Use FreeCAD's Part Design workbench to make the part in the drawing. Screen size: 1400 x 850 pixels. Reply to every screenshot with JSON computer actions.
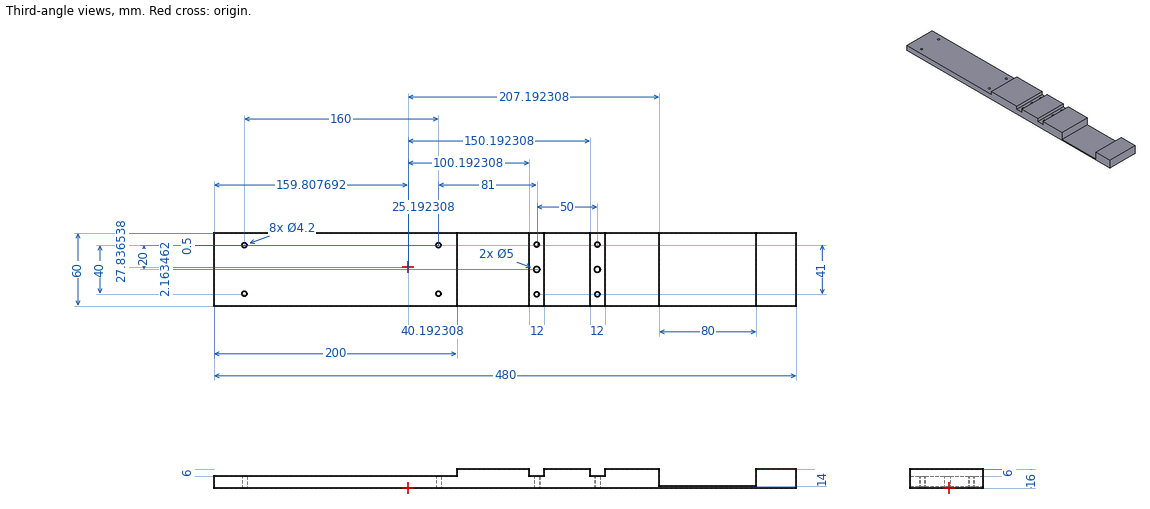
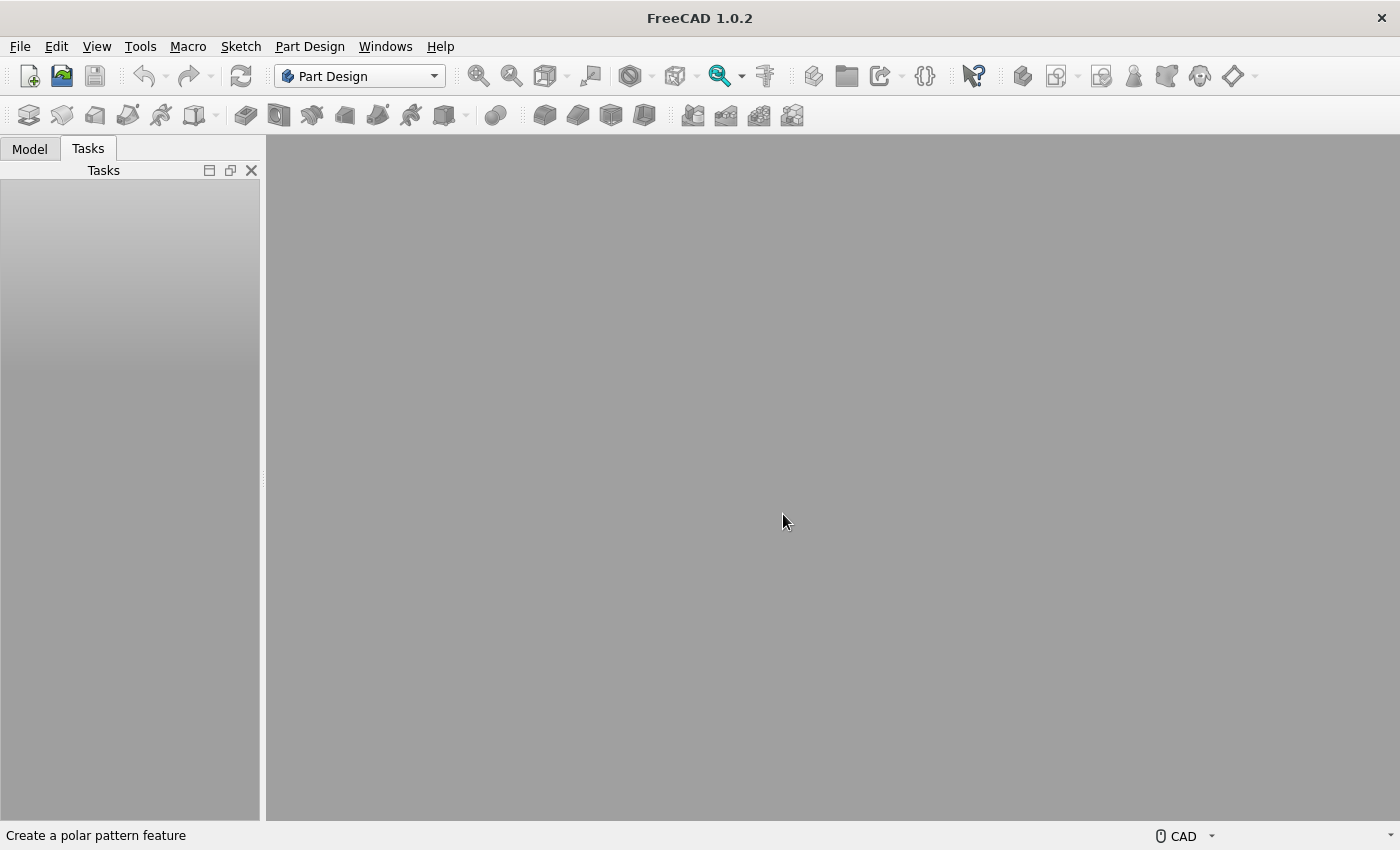
{"action": "left_click", "coordinate": [29, 76]}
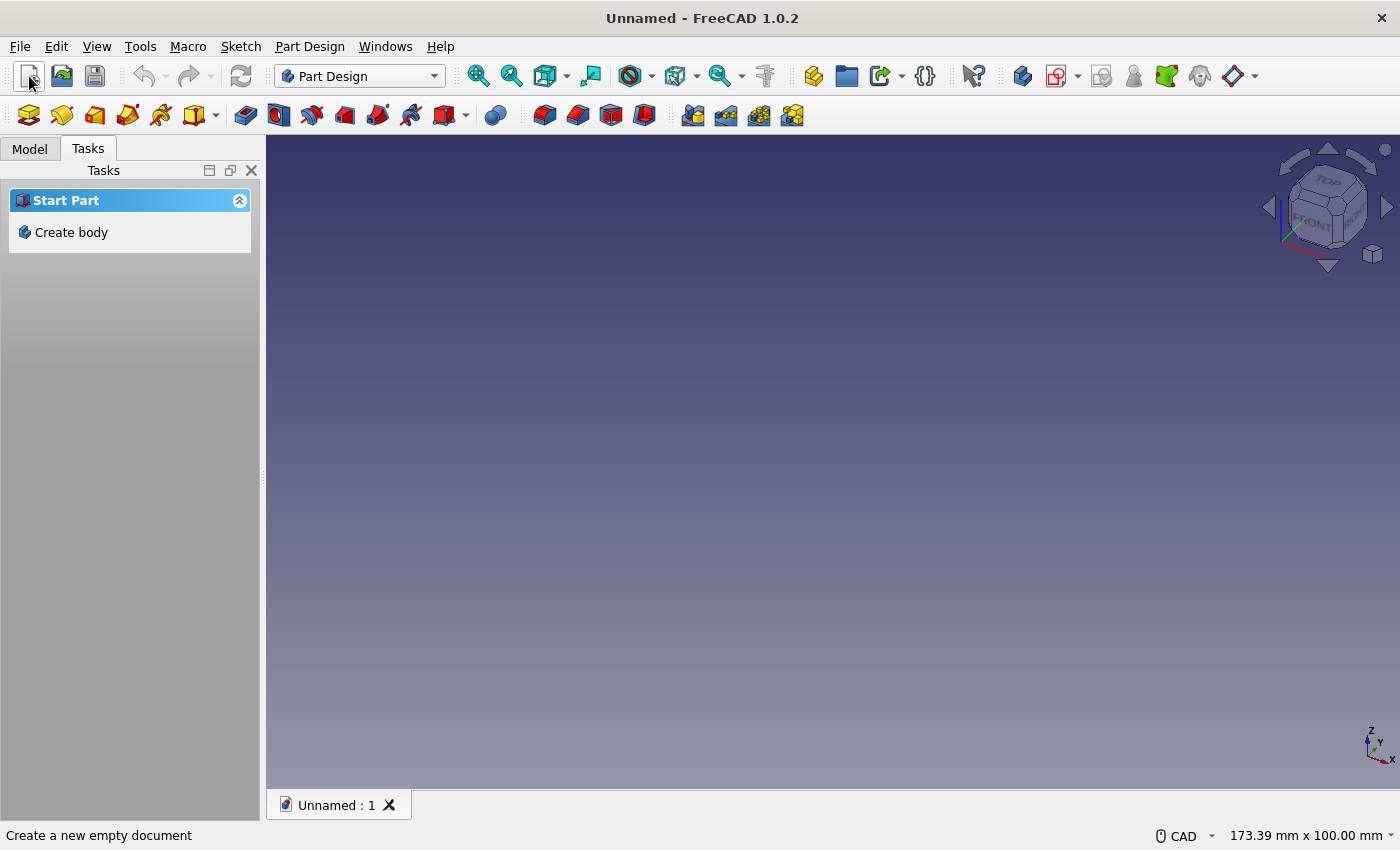
{"action": "left_click", "coordinate": [1056, 76]}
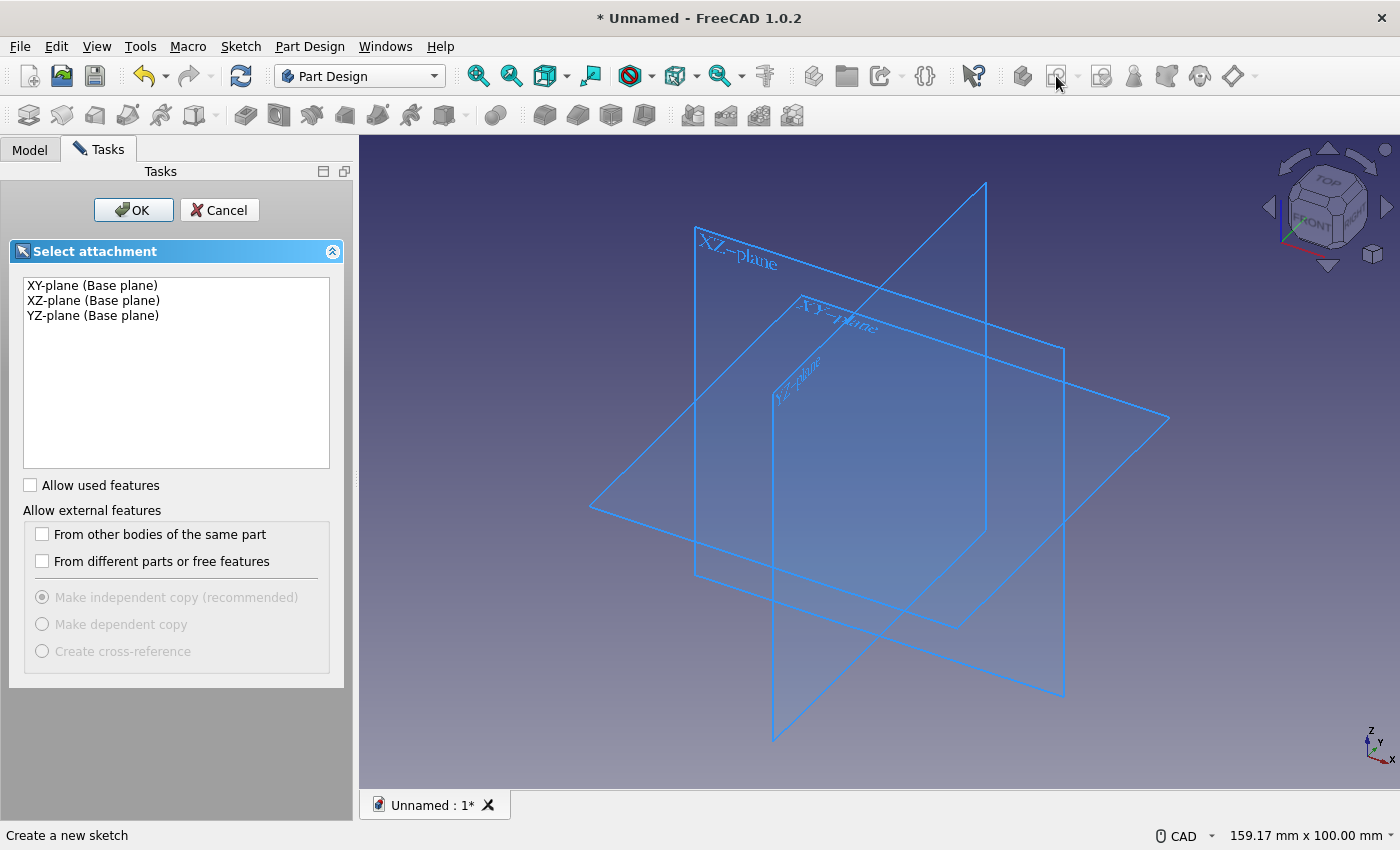
{"action": "left_click", "coordinate": [84, 286]}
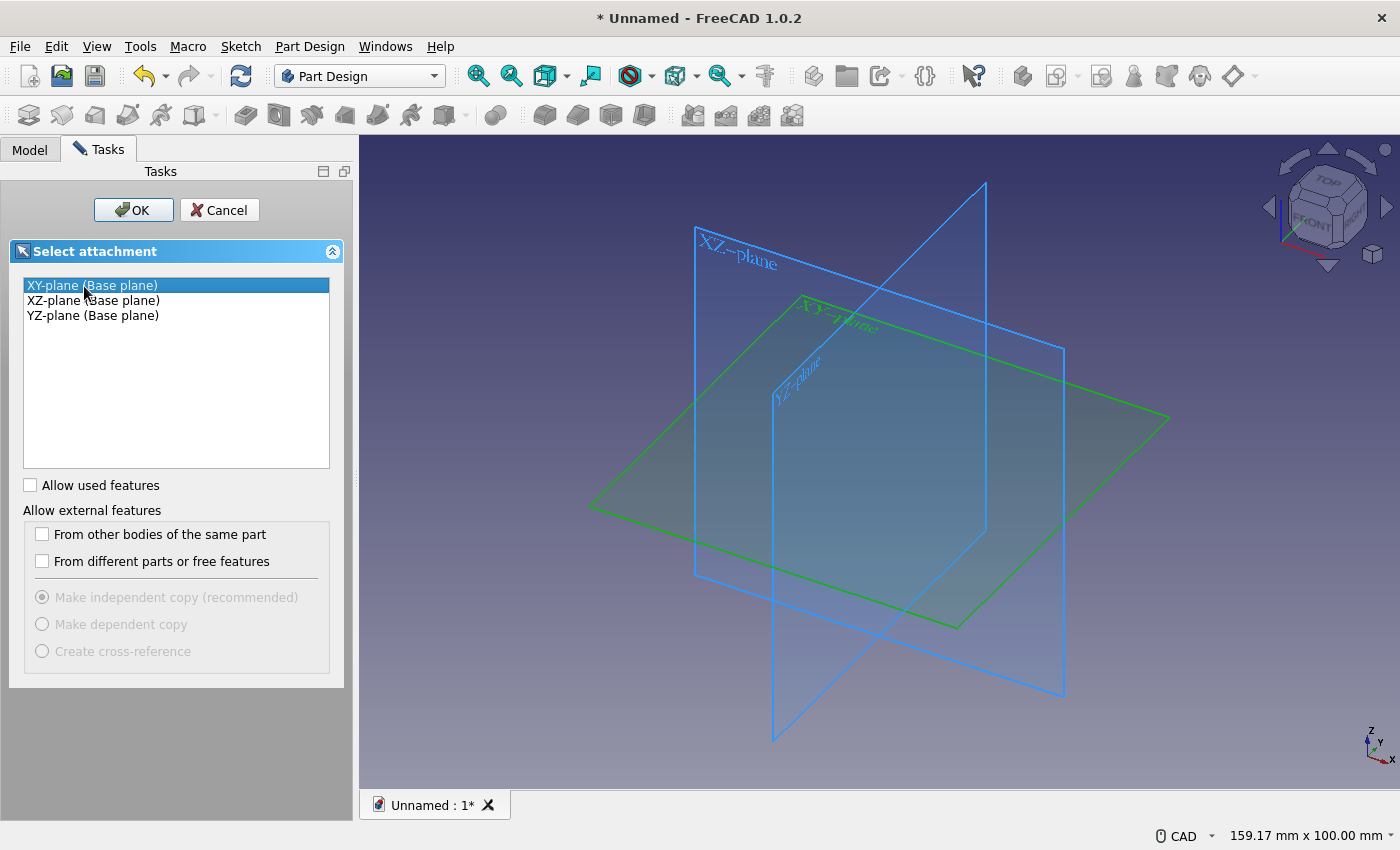
{"action": "left_click", "coordinate": [134, 210]}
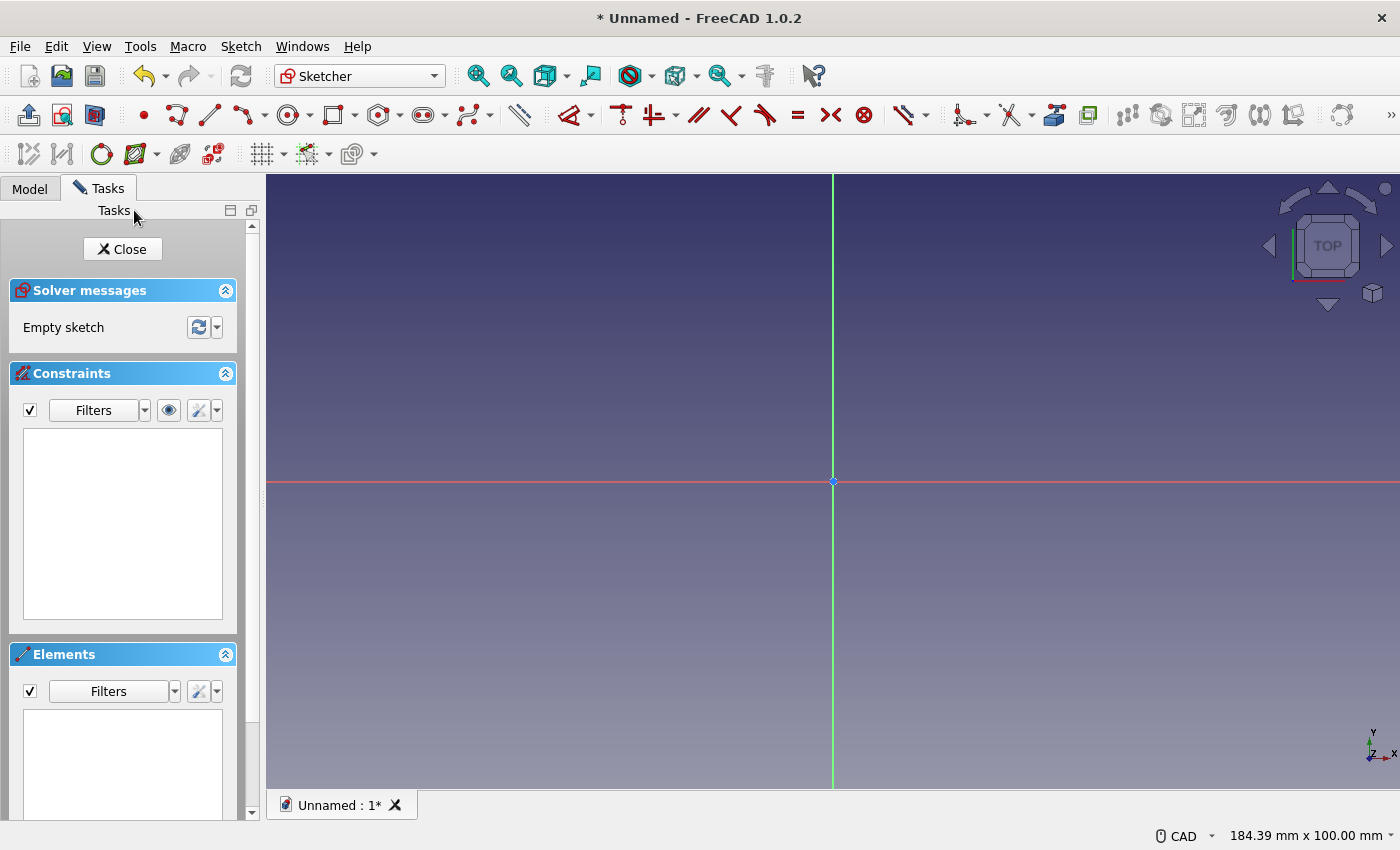
{"action": "scroll", "coordinate": [581, 477], "scroll_direction": "down", "scroll_amount": 7}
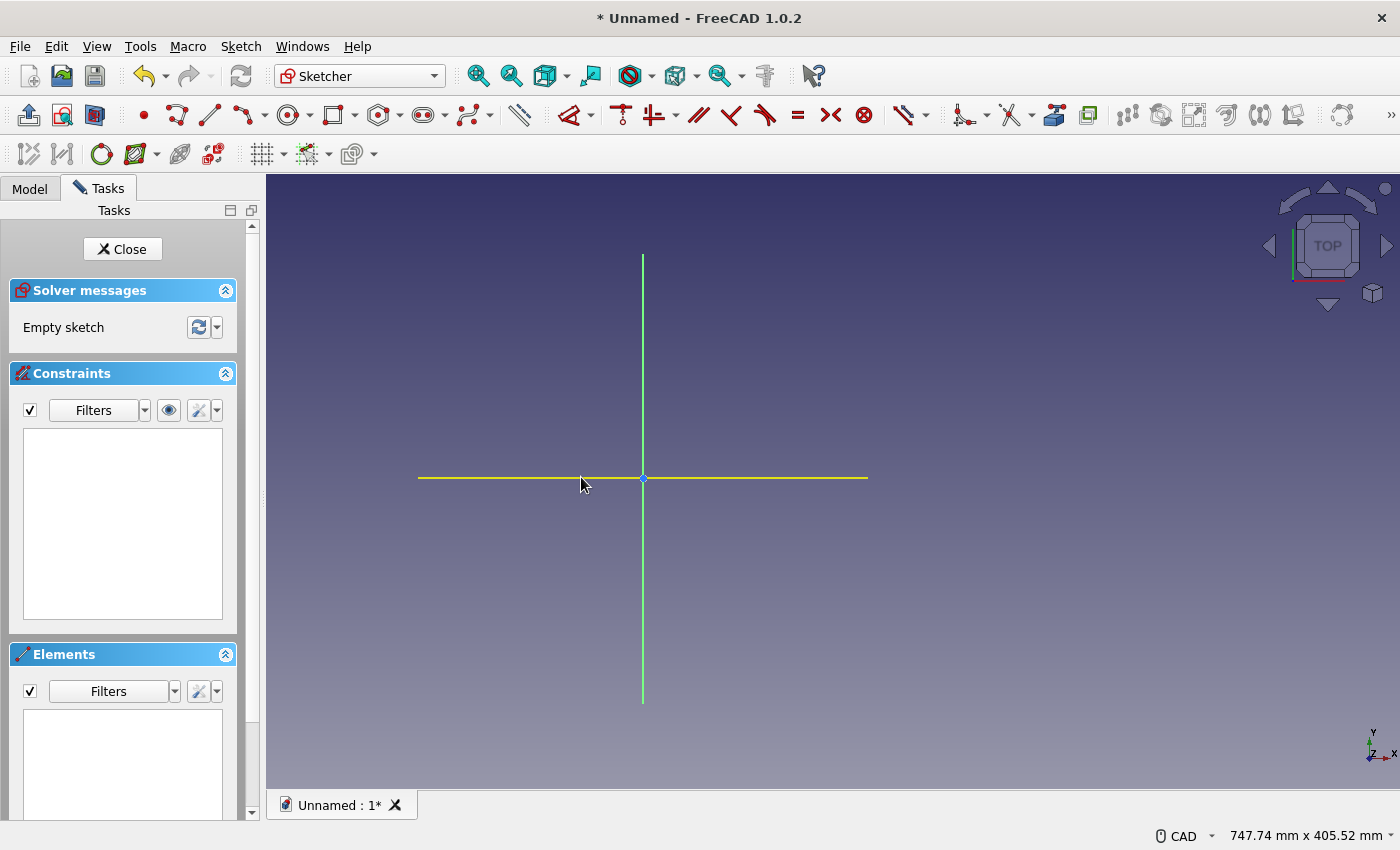
{"action": "left_click", "coordinate": [332, 116]}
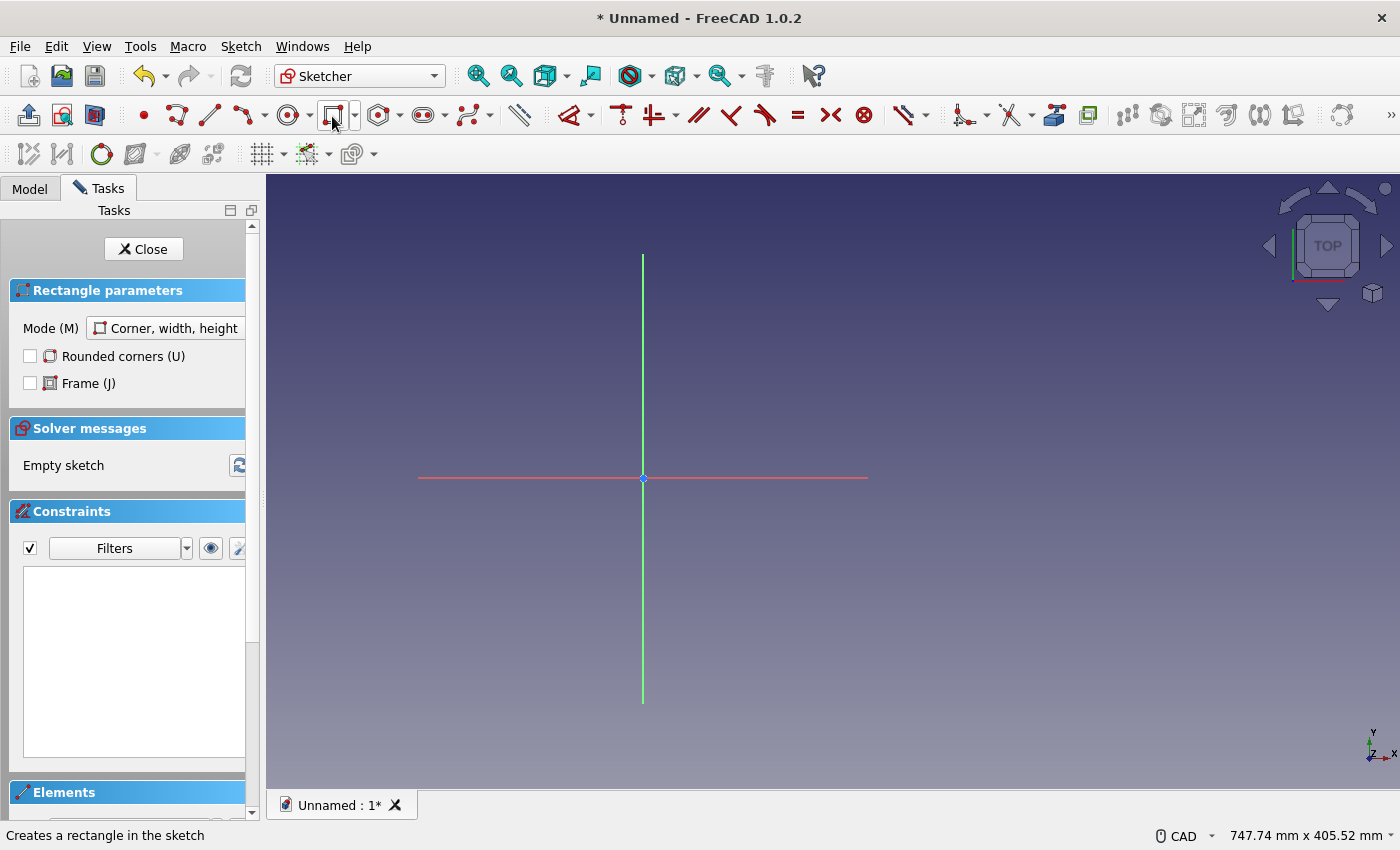
{"action": "left_click", "coordinate": [401, 436]}
{"action": "left_click", "coordinate": [1129, 527]}
{"action": "key", "text": "Escape"}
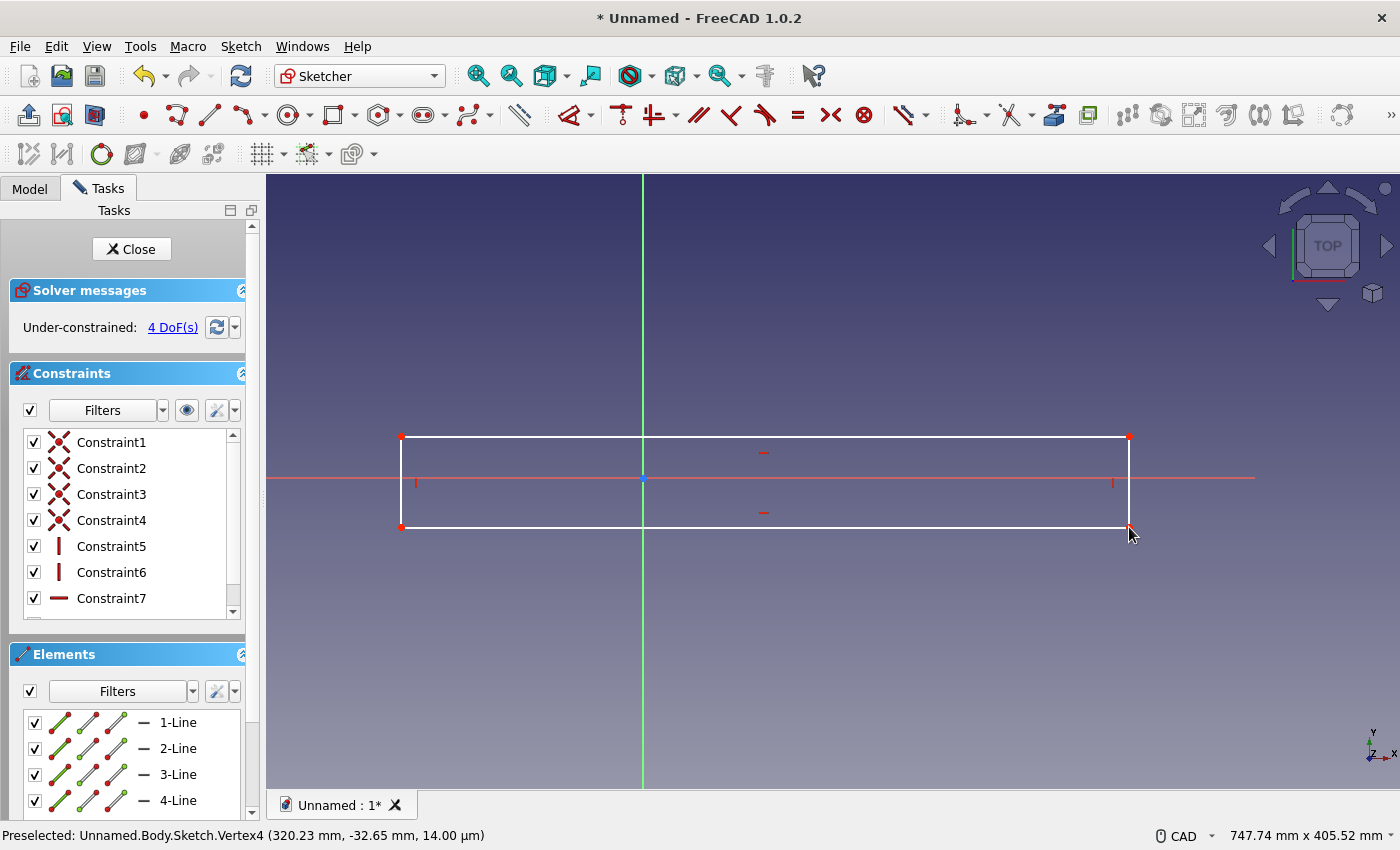
{"action": "left_click", "coordinate": [568, 116]}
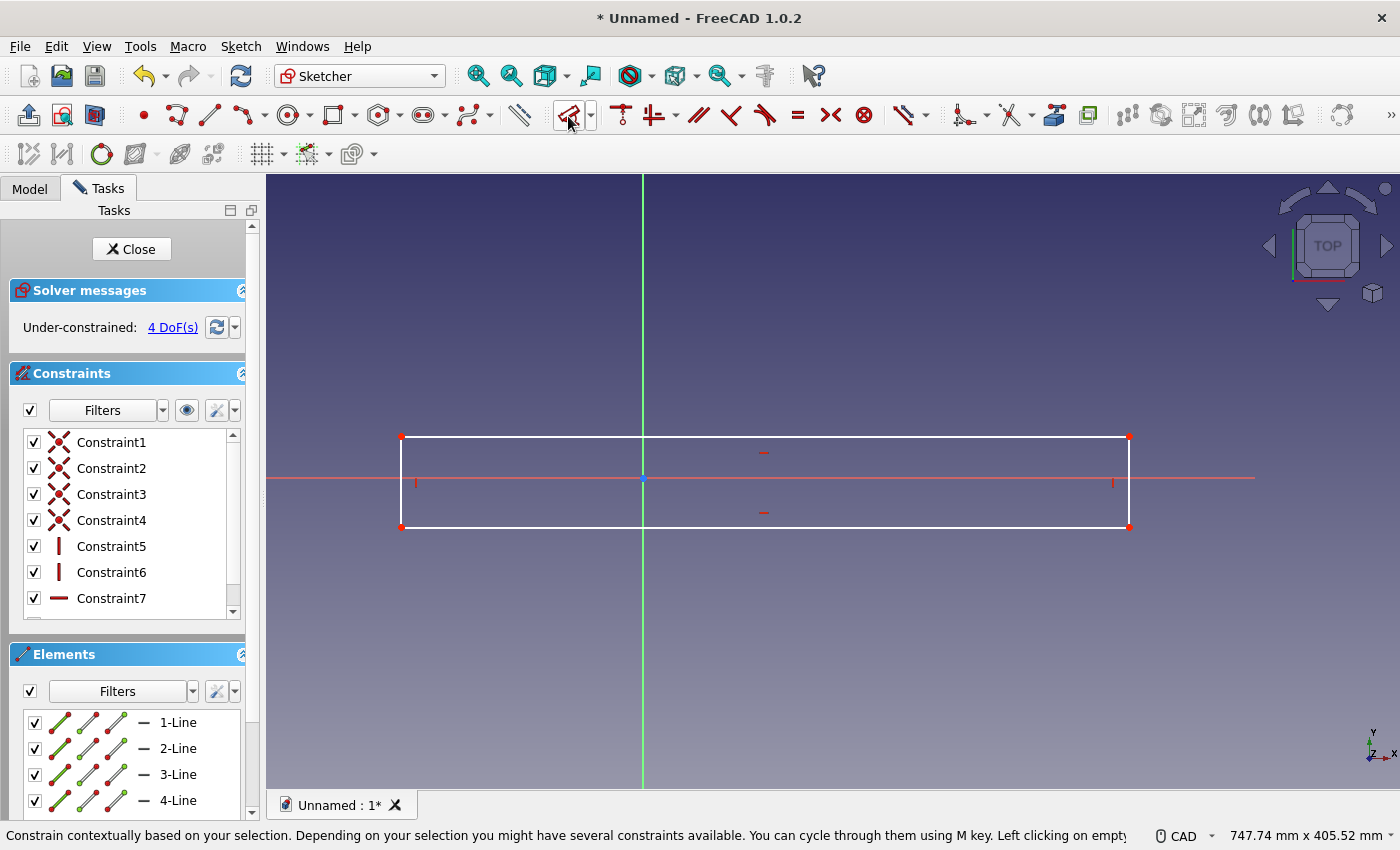
{"action": "left_click", "coordinate": [401, 464]}
{"action": "left_click", "coordinate": [367, 462]}